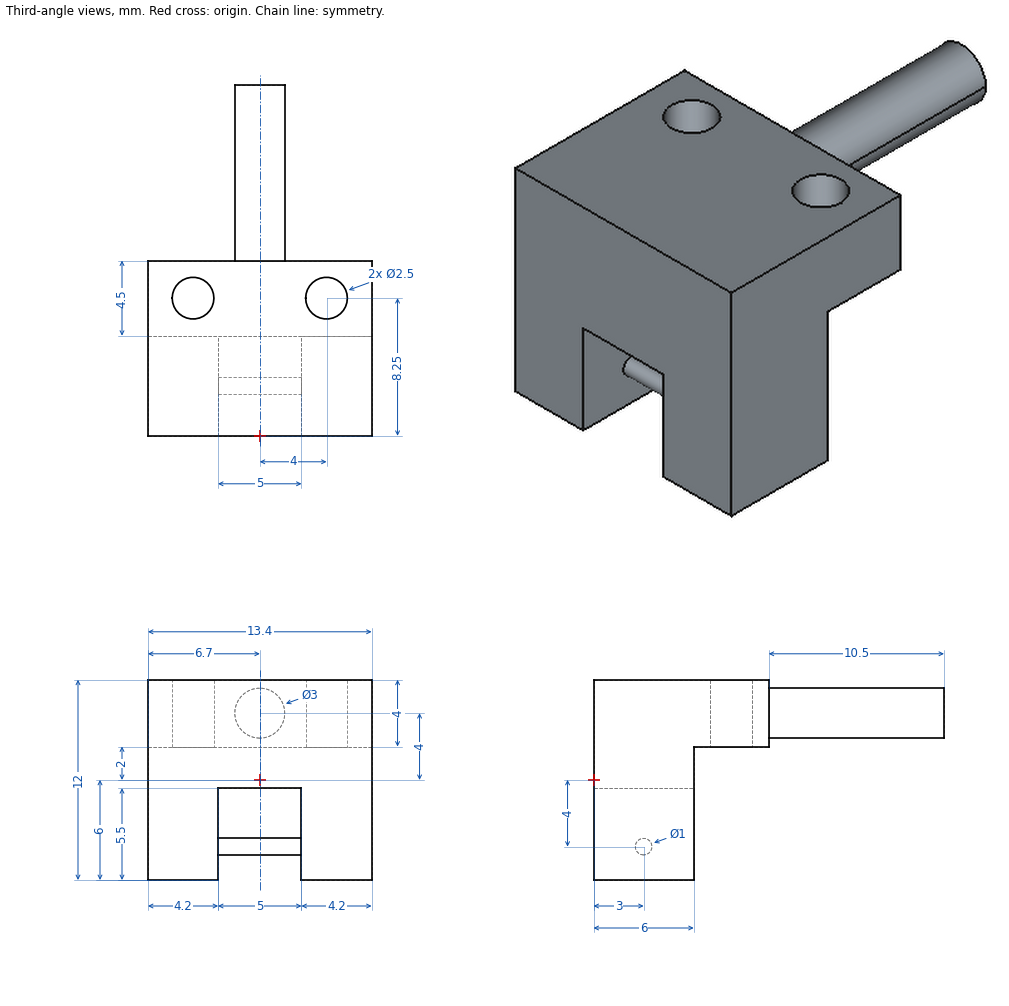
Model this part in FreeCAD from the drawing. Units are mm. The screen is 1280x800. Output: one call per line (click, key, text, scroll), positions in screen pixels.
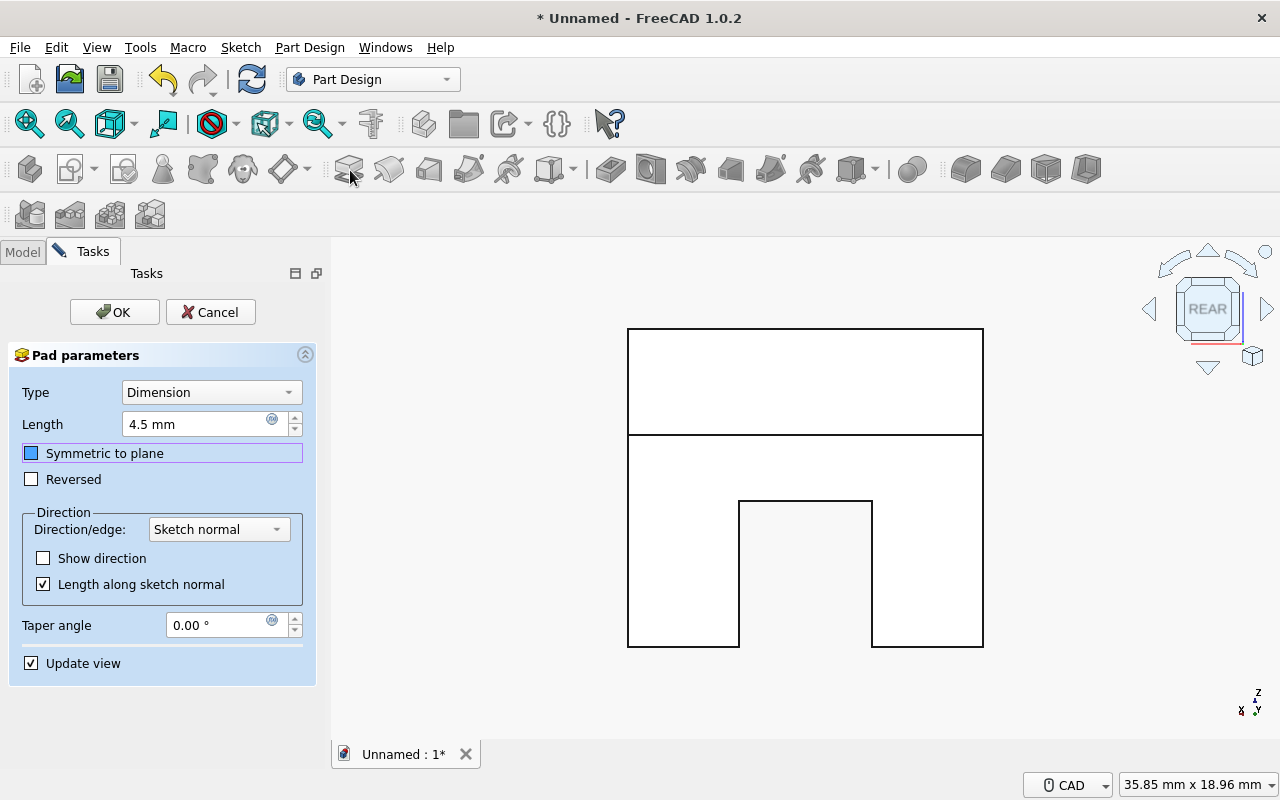
click(115, 312)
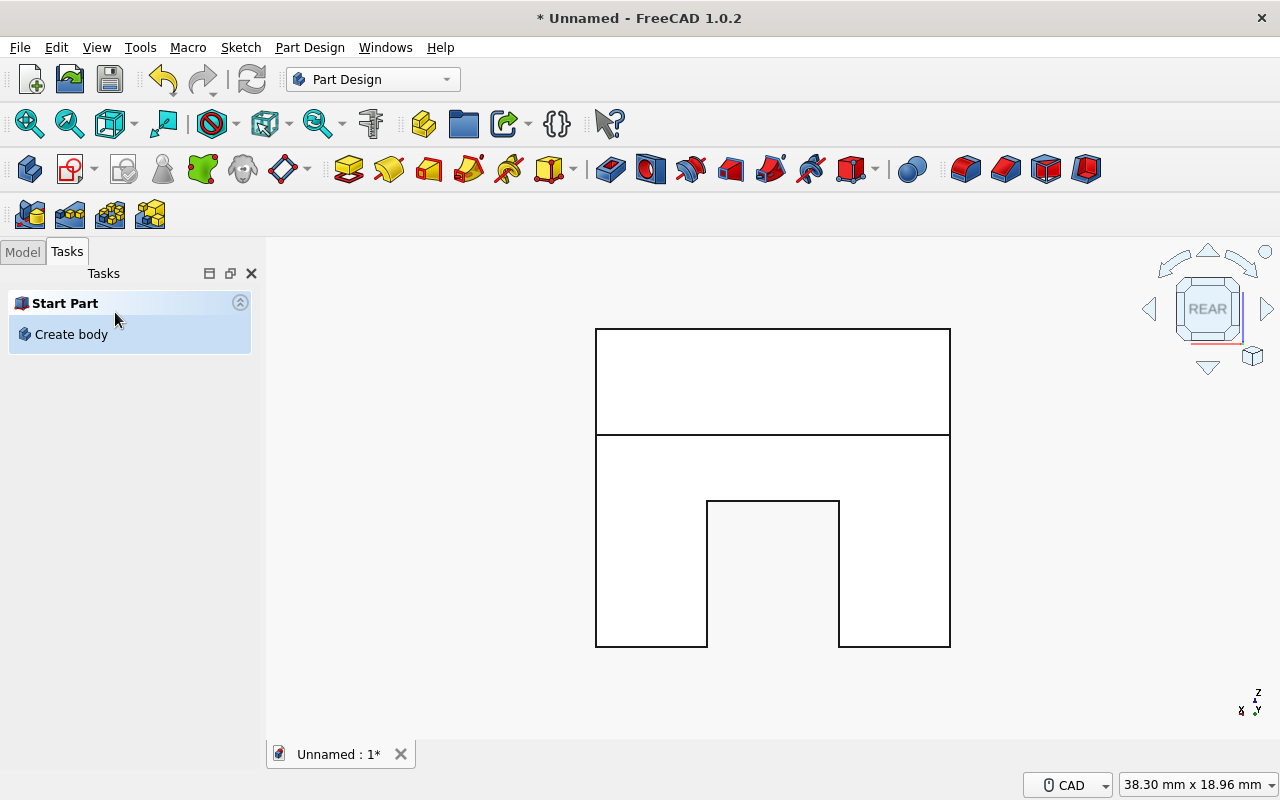
click(672, 381)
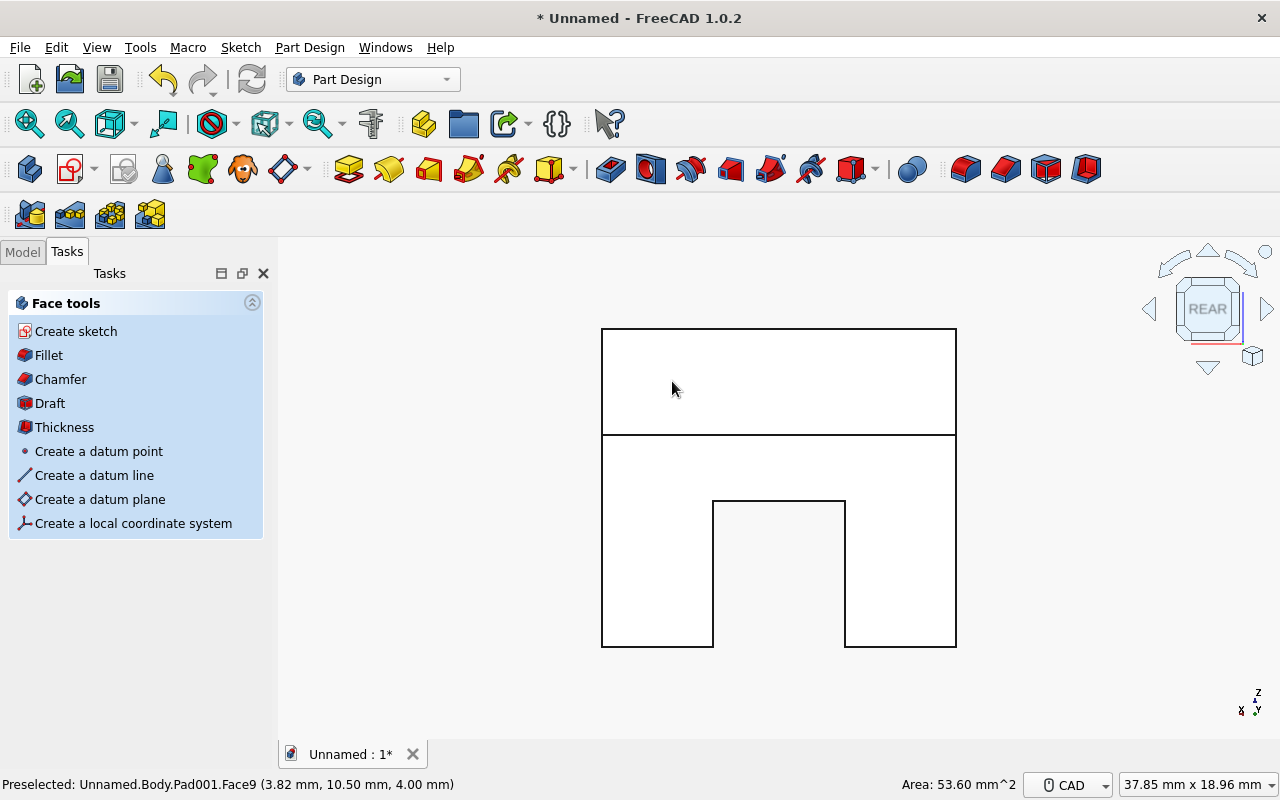
click(70, 170)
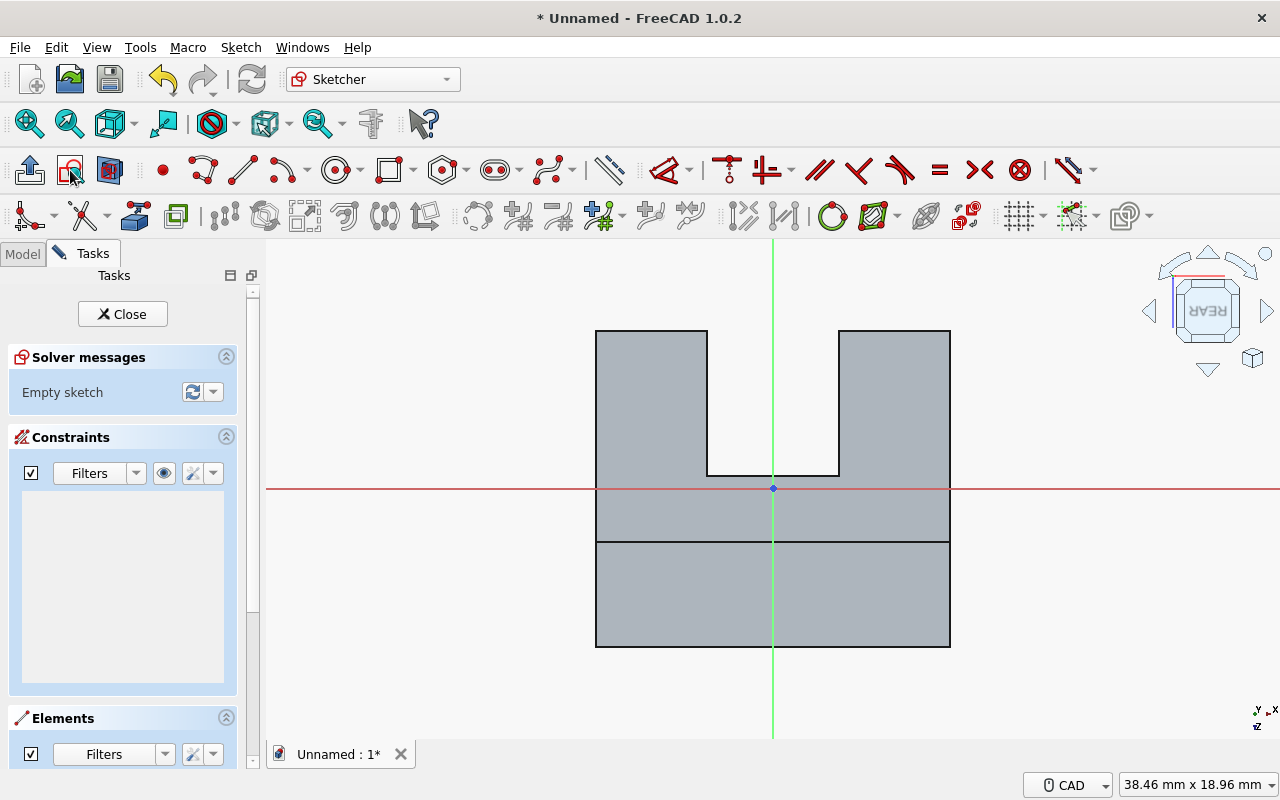
scroll(829, 621, up, 4)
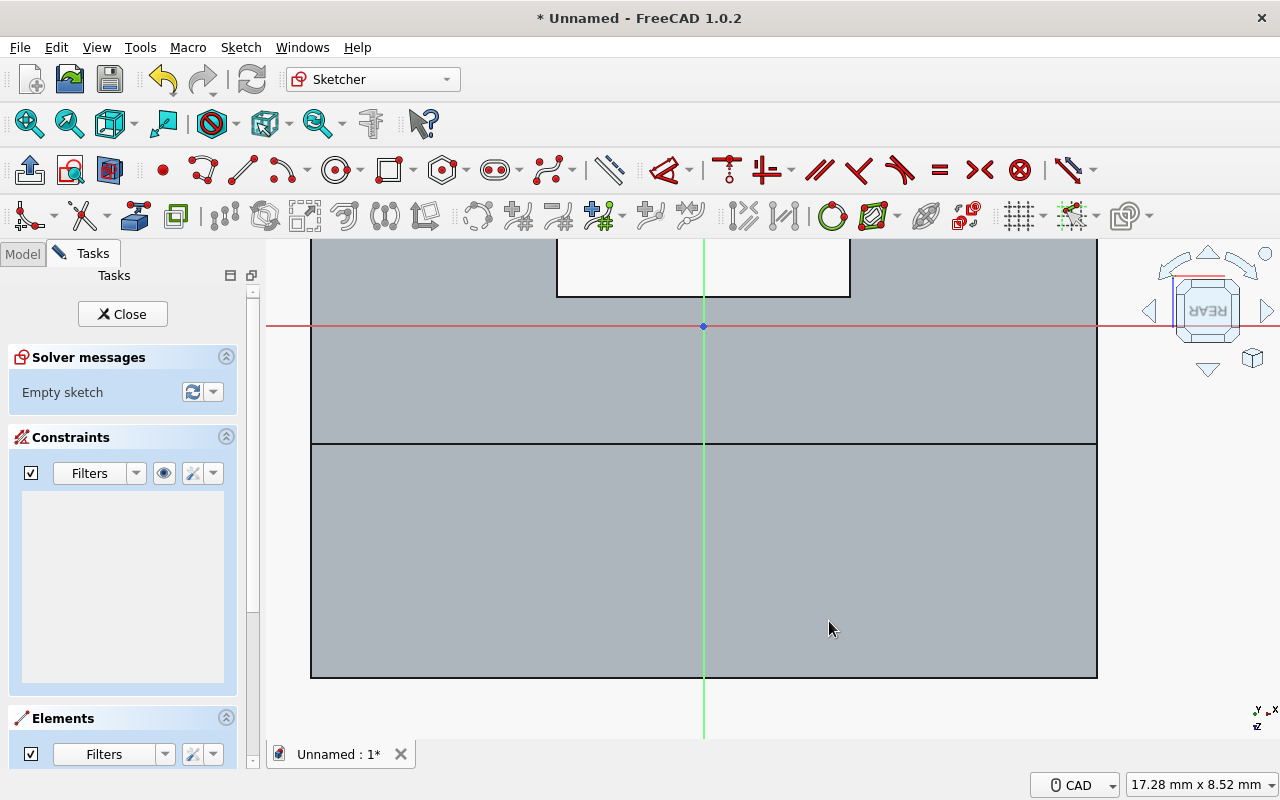
click(336, 170)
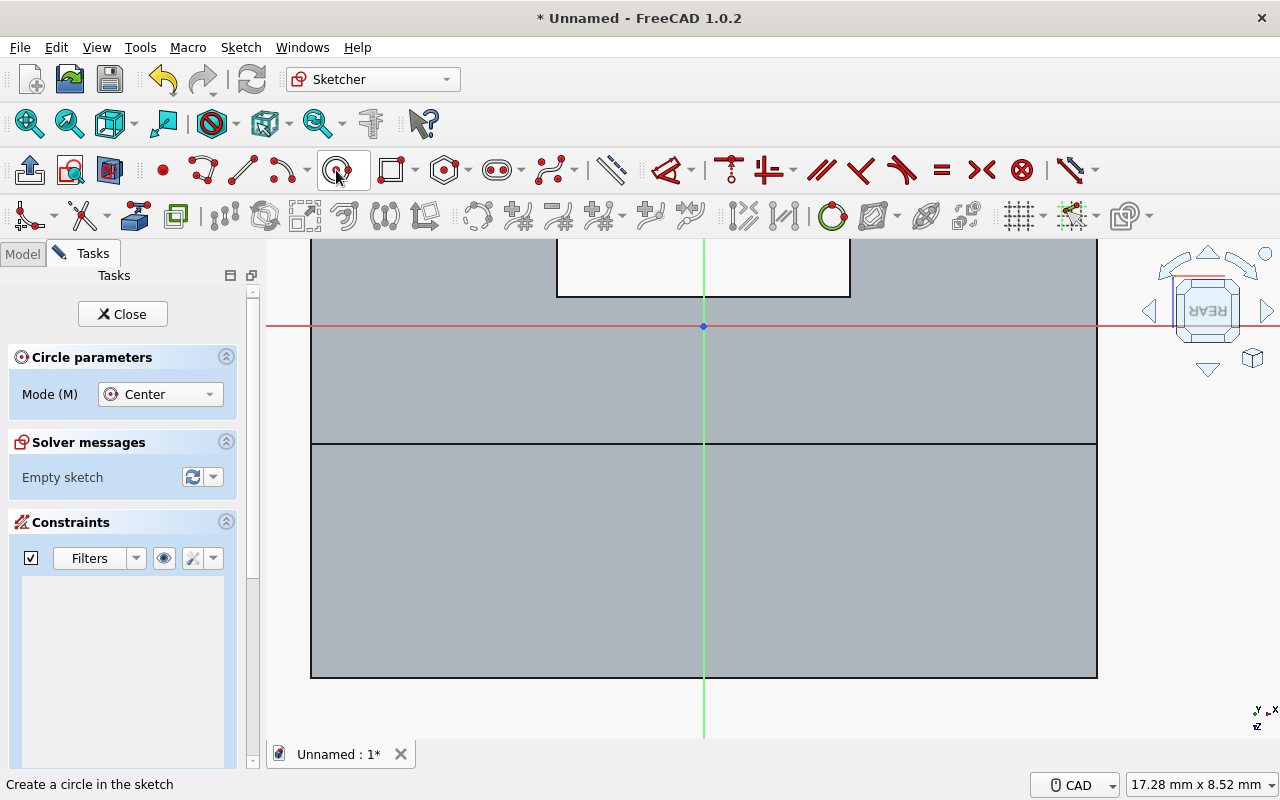
click(704, 561)
move(766, 499)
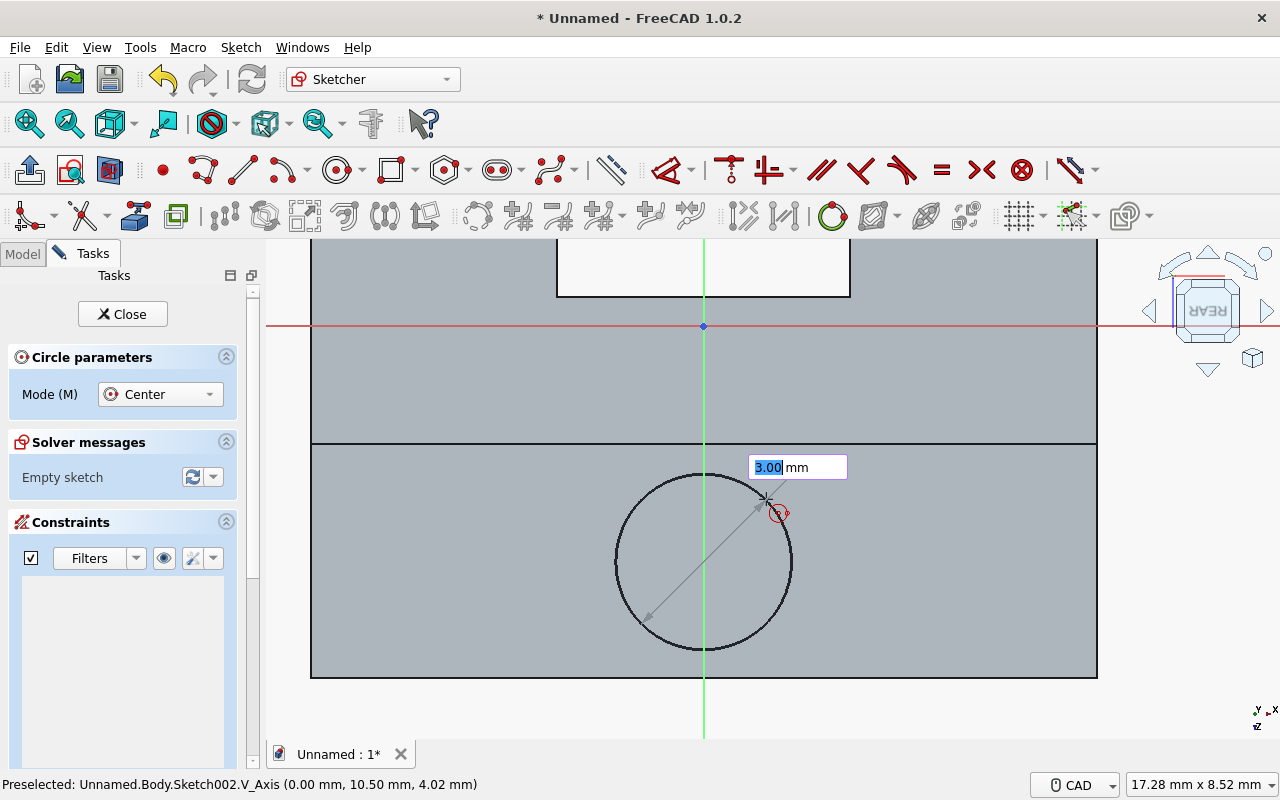
text(3)
key(Return)
key(Escape)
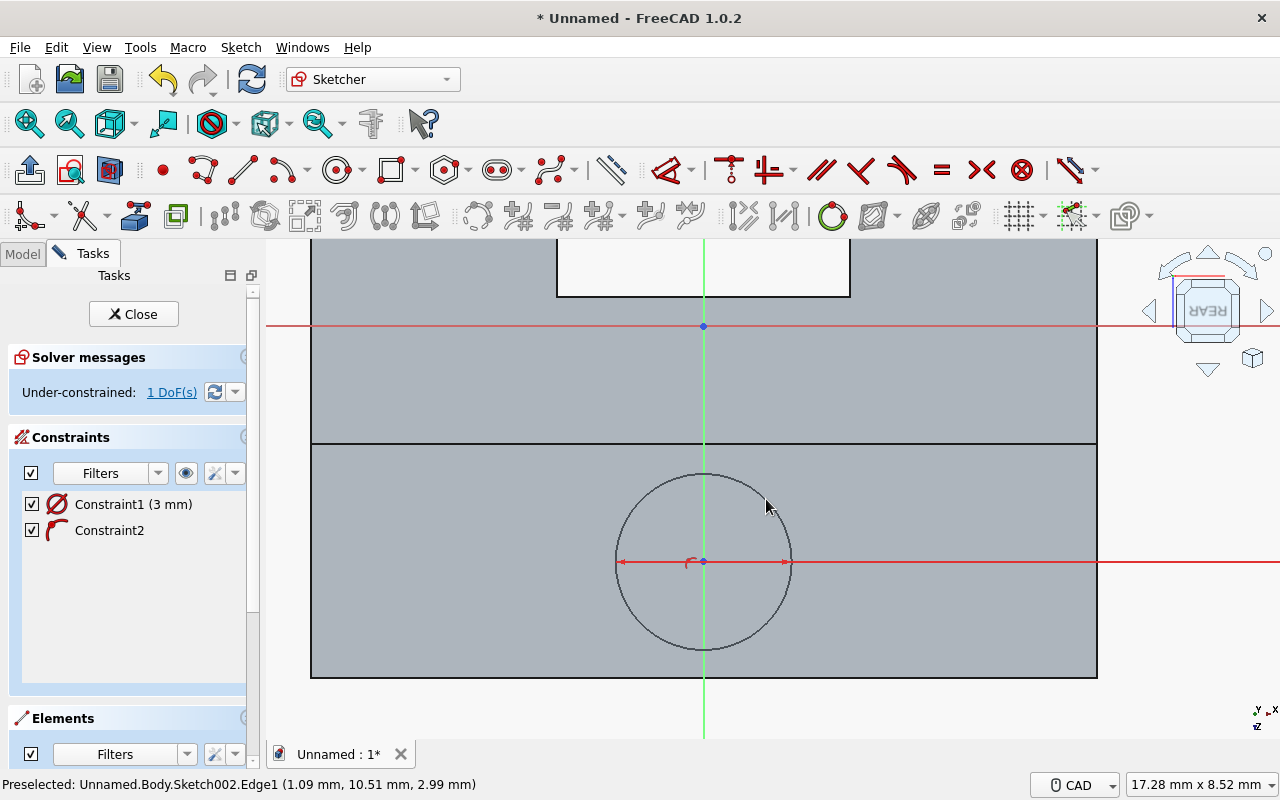
click(666, 170)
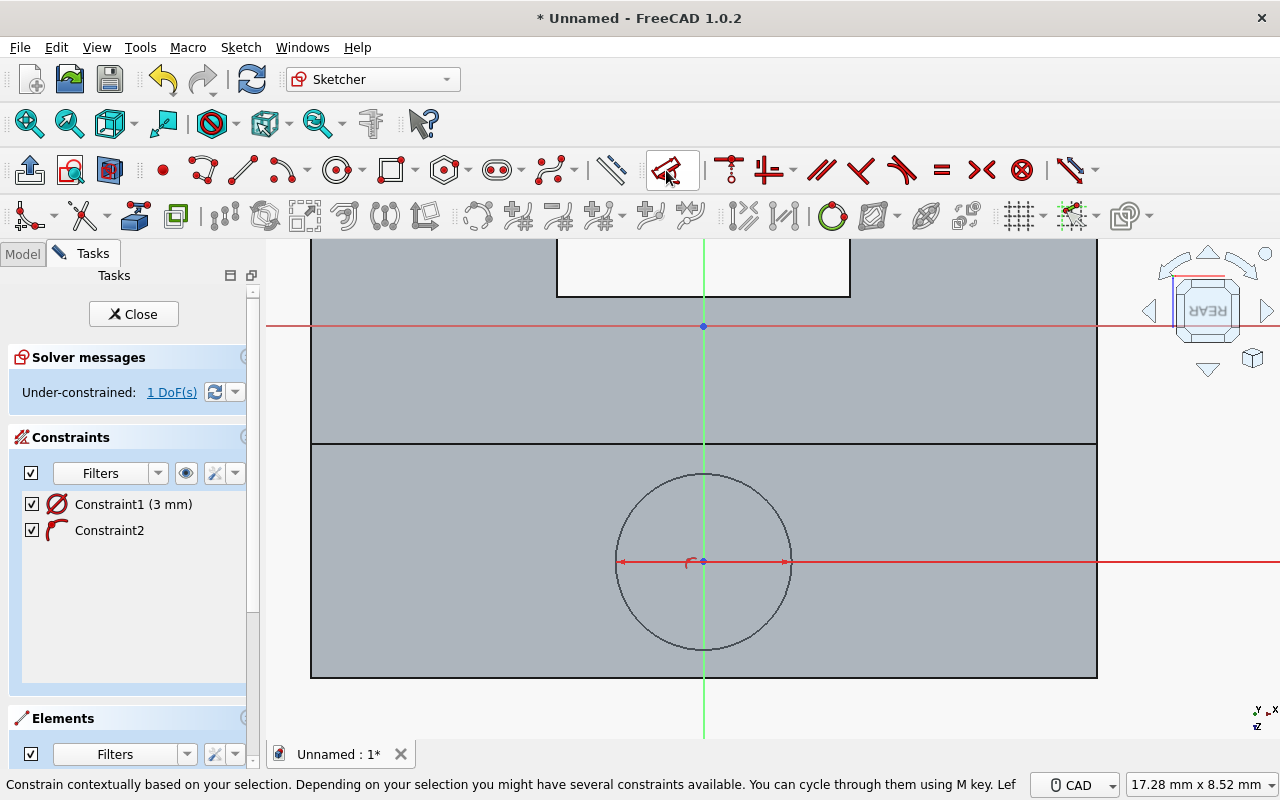
click(704, 562)
click(738, 444)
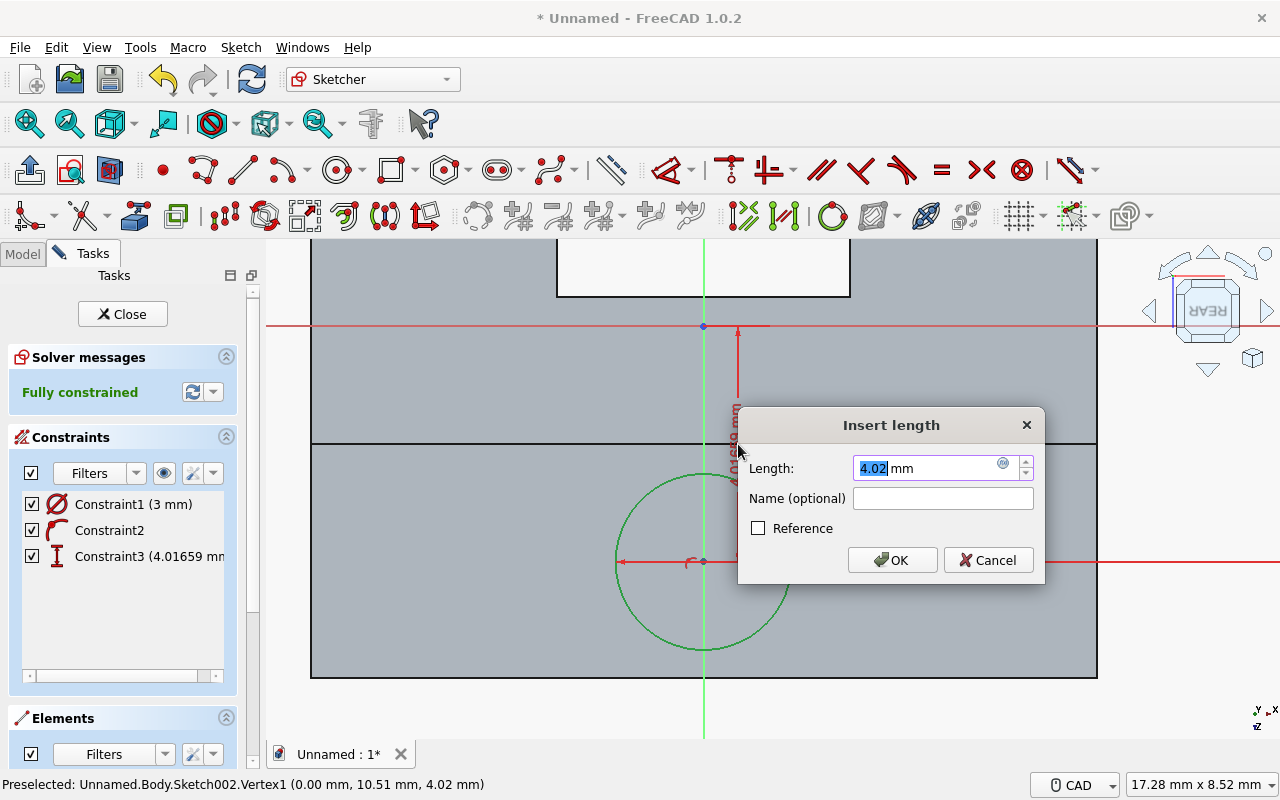
text(4)
key(Return)
key(Escape)